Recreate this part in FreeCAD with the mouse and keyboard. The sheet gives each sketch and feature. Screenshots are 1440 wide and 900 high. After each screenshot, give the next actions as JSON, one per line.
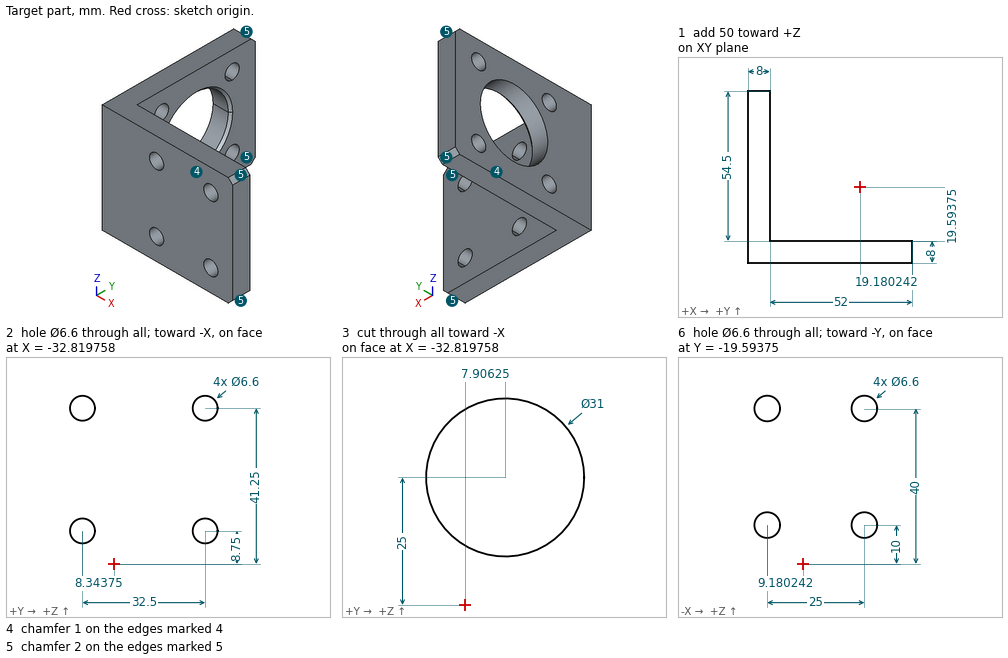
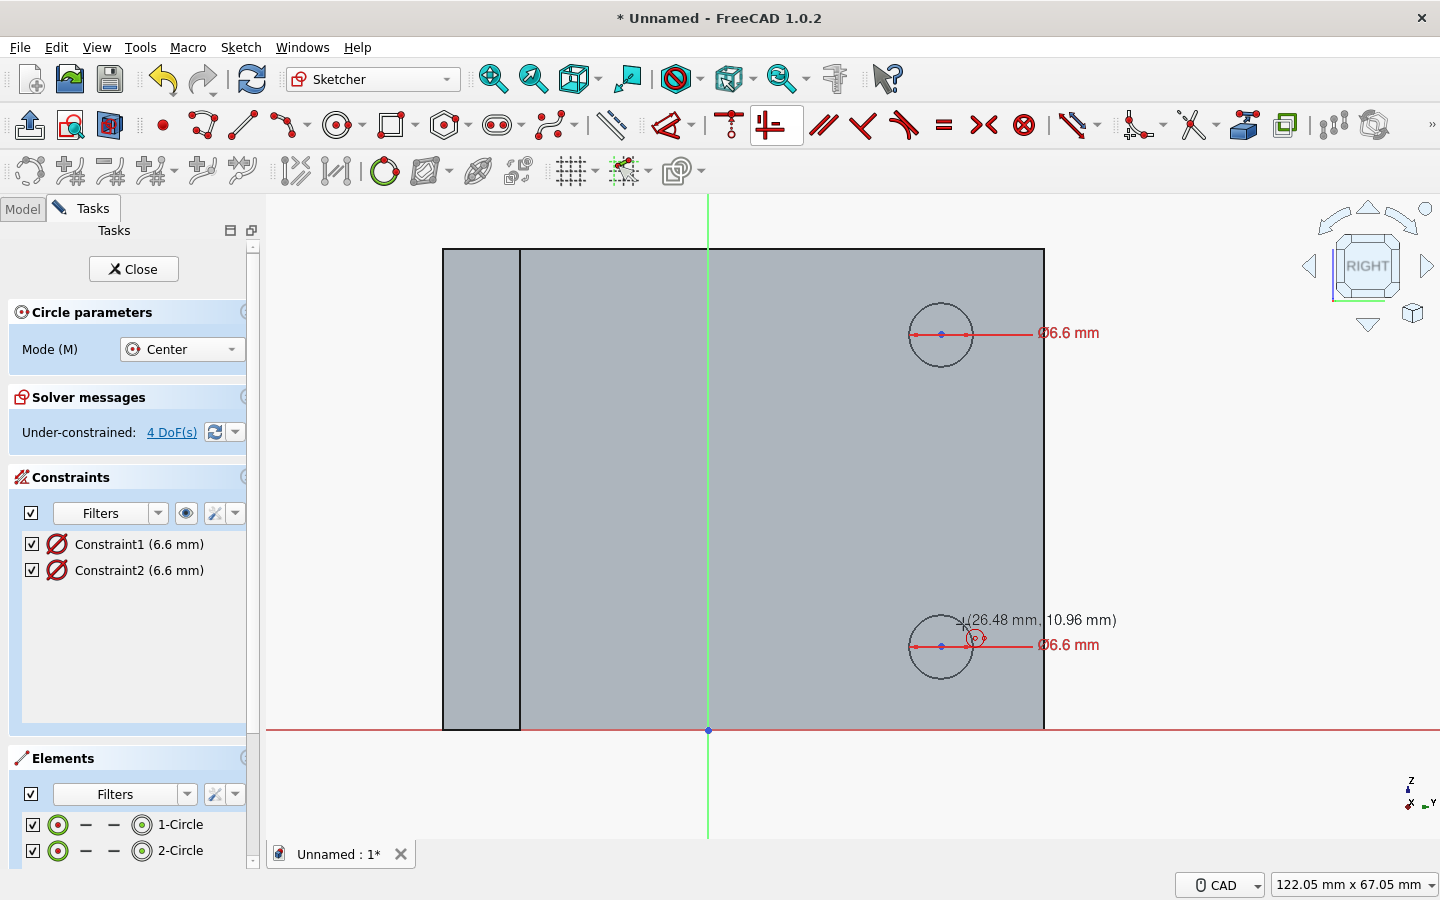
{"action": "left_click", "coordinate": [628, 646]}
{"action": "mouse_move", "coordinate": [650, 624]}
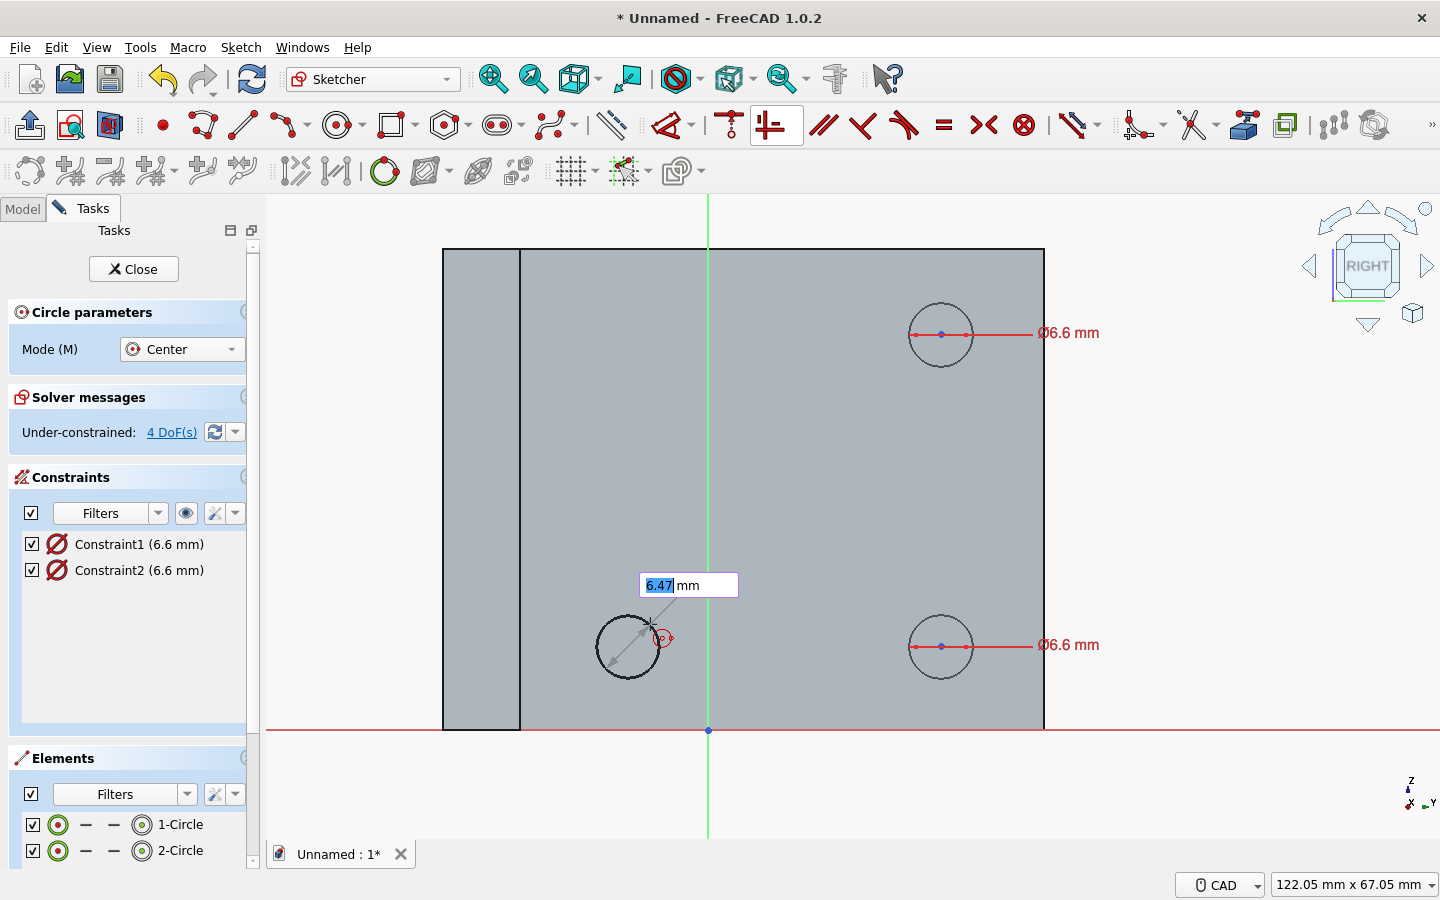
{"action": "type", "text": "6.6"}
{"action": "key", "text": "Return"}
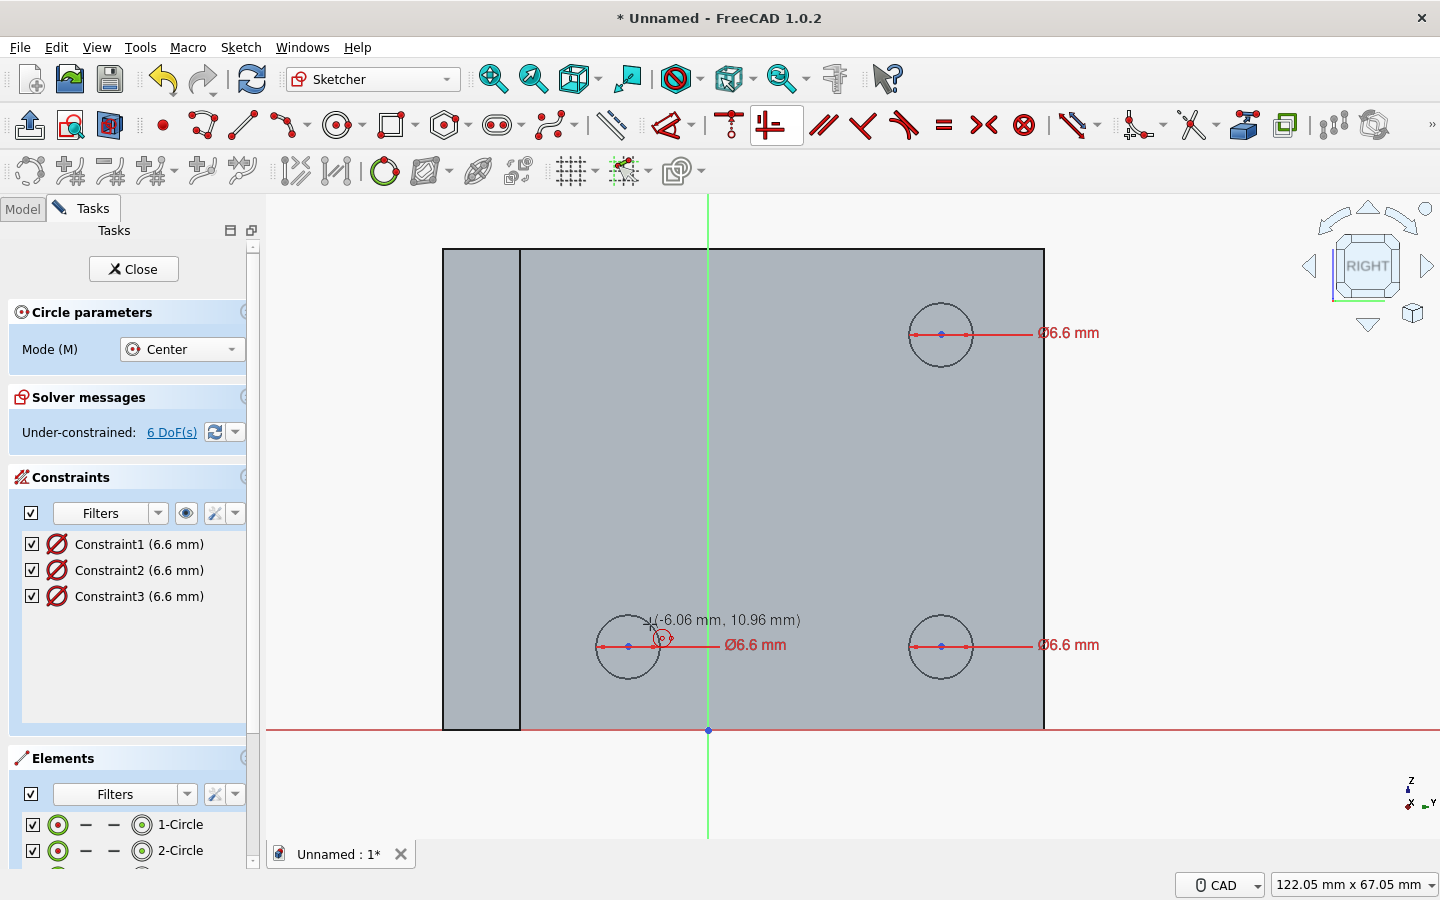
{"action": "left_click", "coordinate": [628, 334]}
{"action": "mouse_move", "coordinate": [650, 311]}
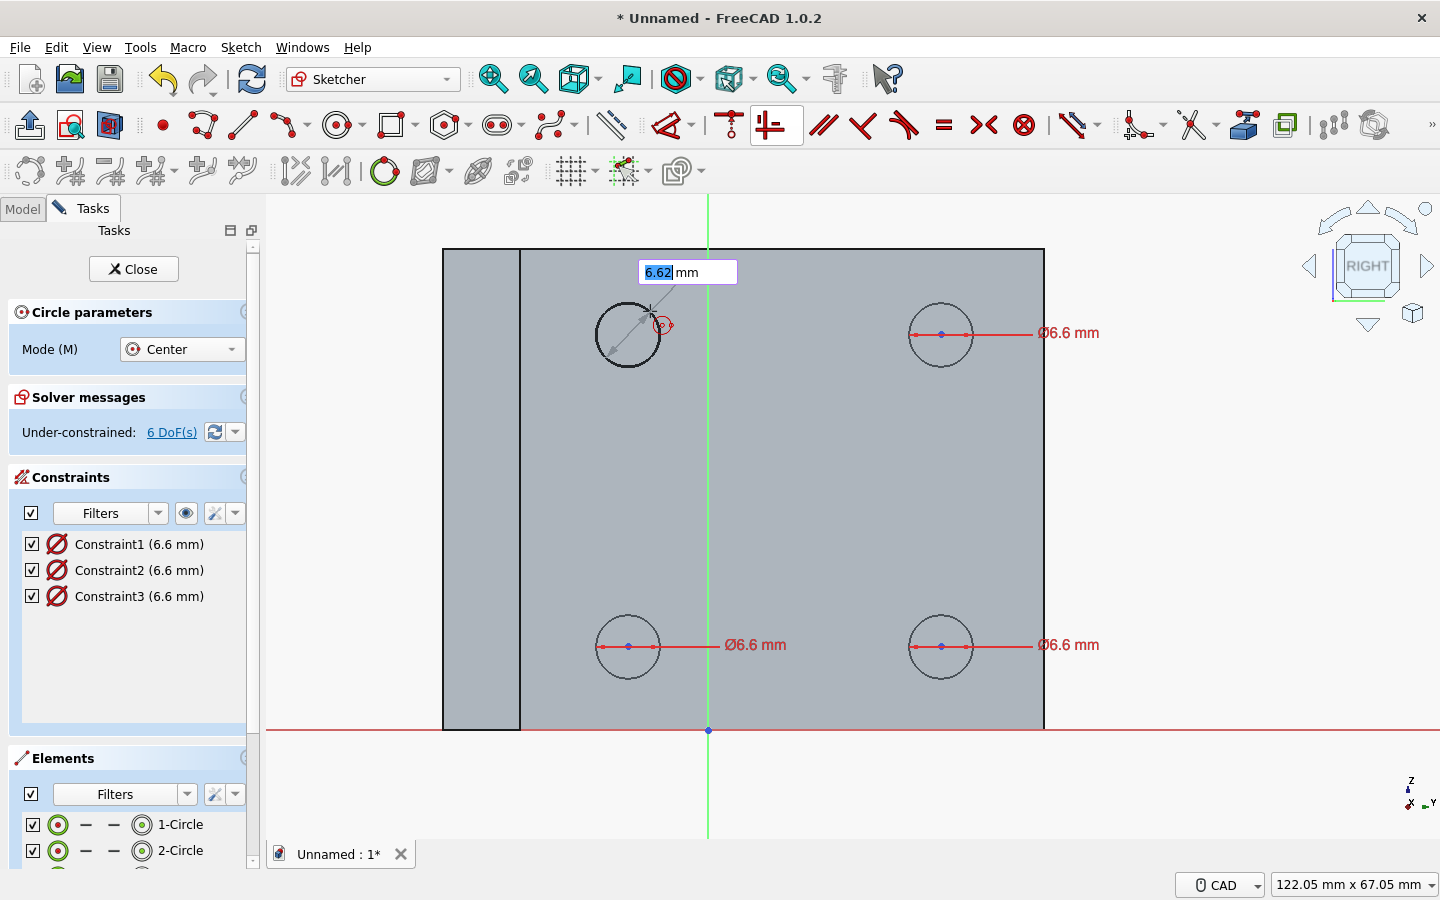
{"action": "type", "text": "6.6"}
{"action": "key", "text": "Return"}
{"action": "key", "text": "Escape"}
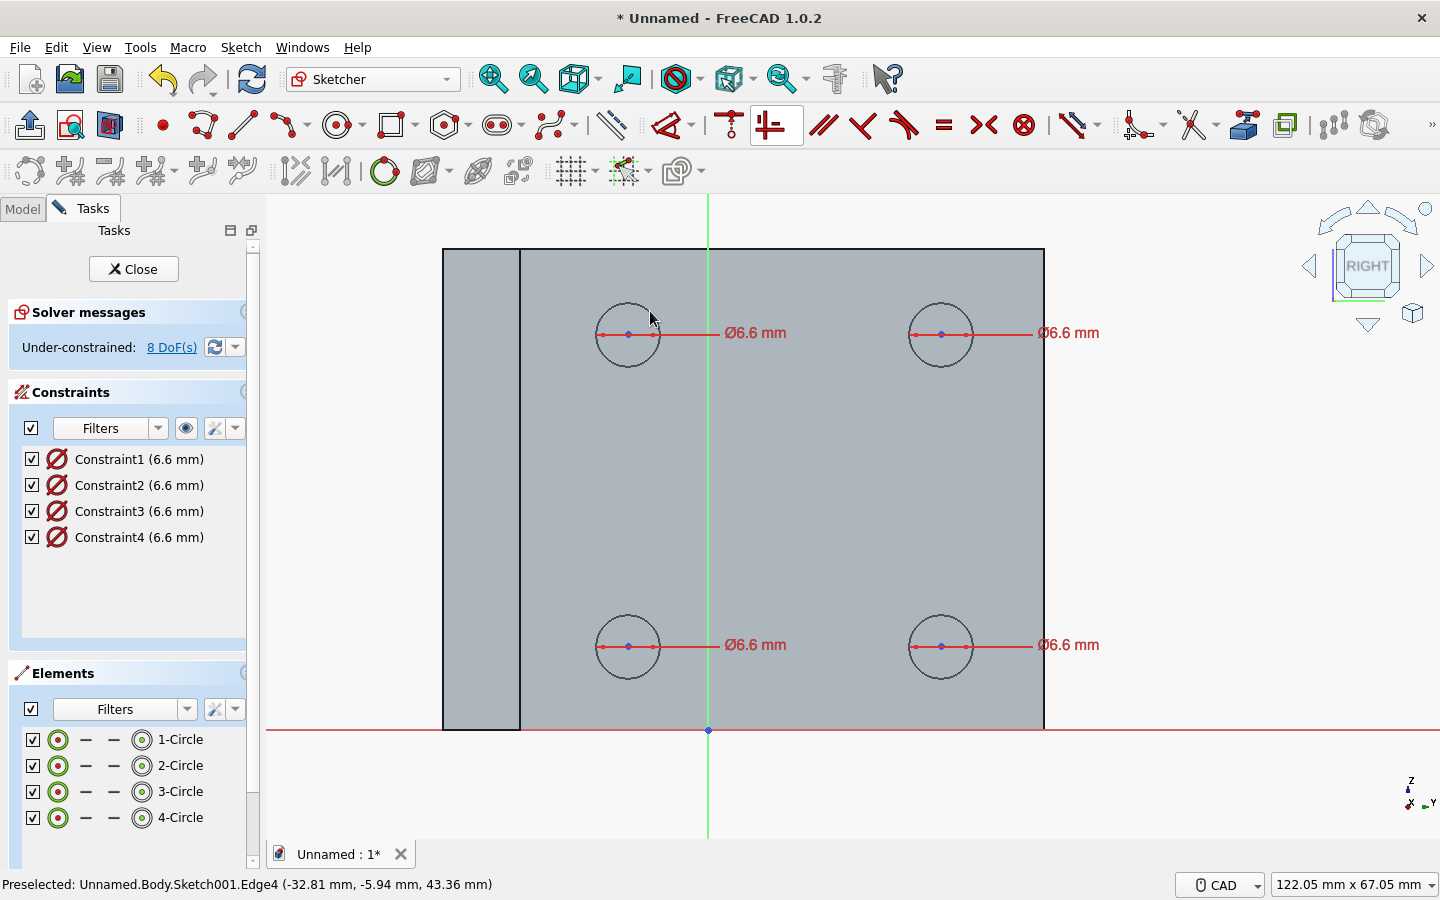
{"action": "left_click", "coordinate": [941, 335]}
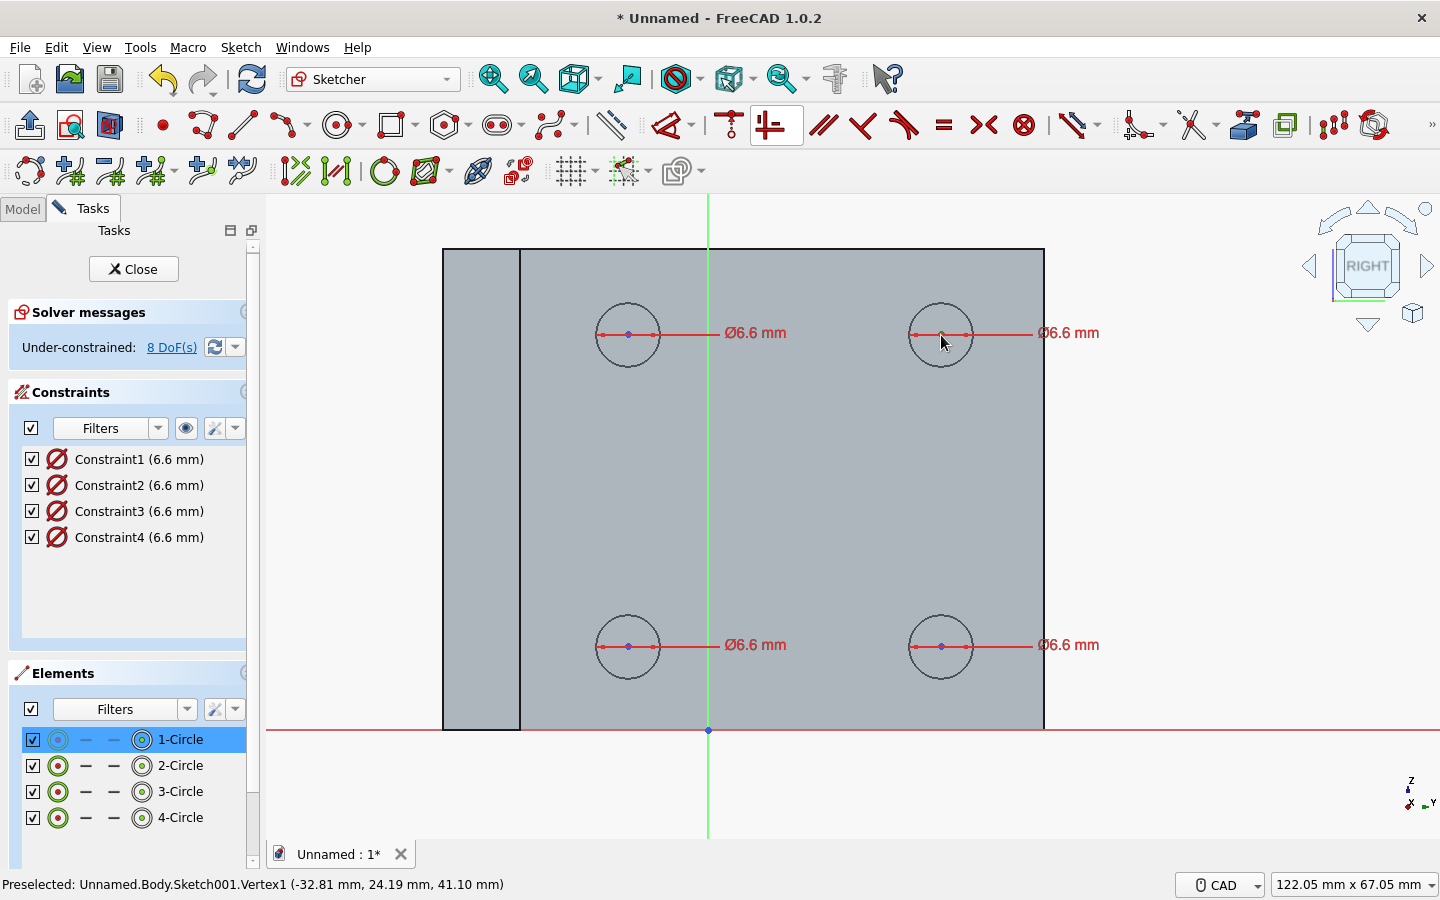
{"action": "left_click", "coordinate": [941, 647]}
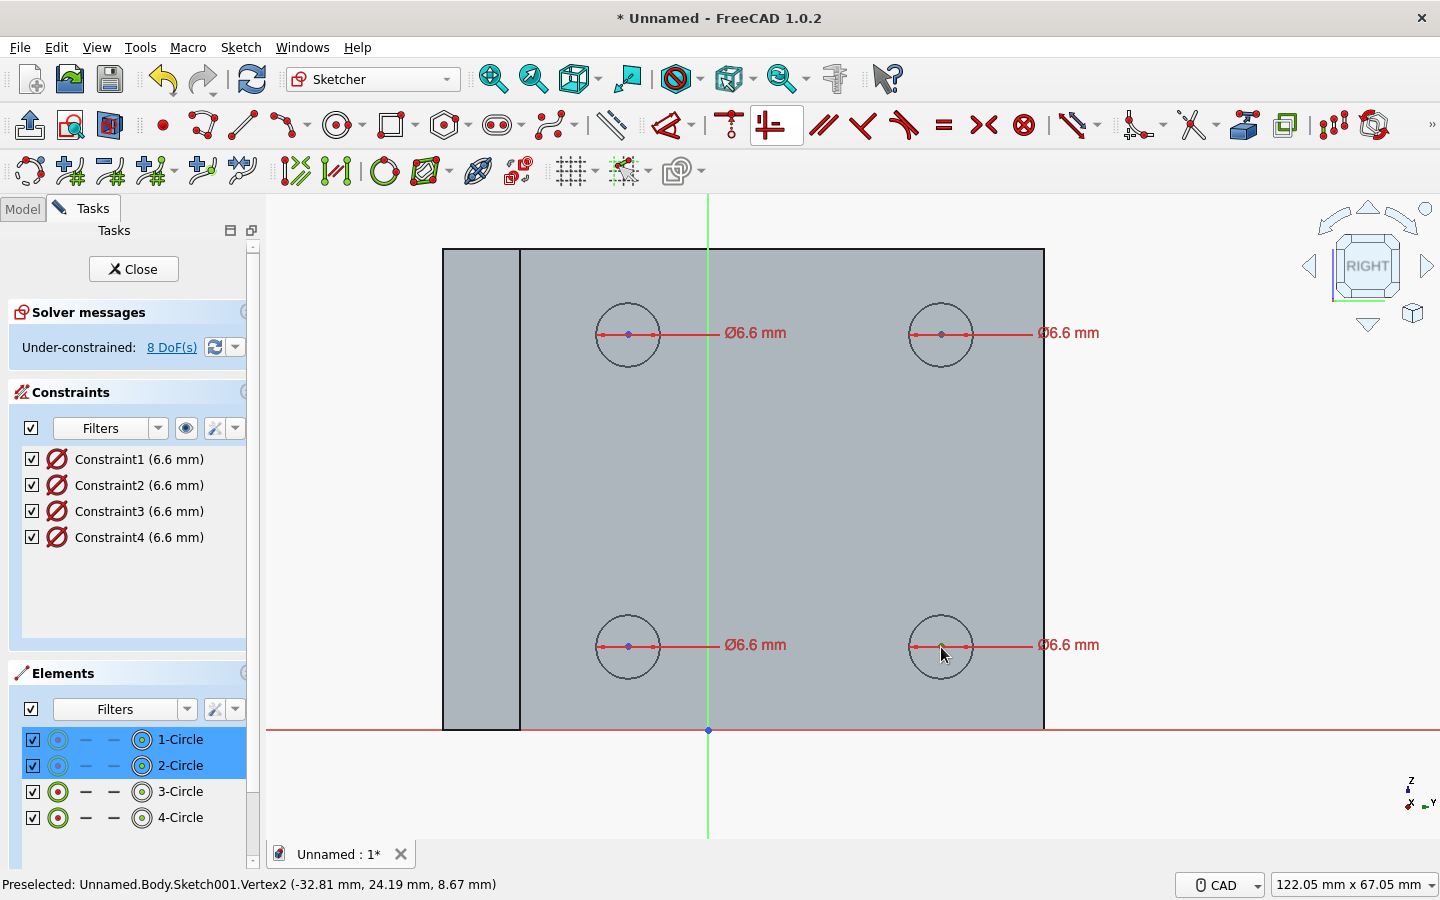
{"action": "left_click", "coordinate": [798, 126]}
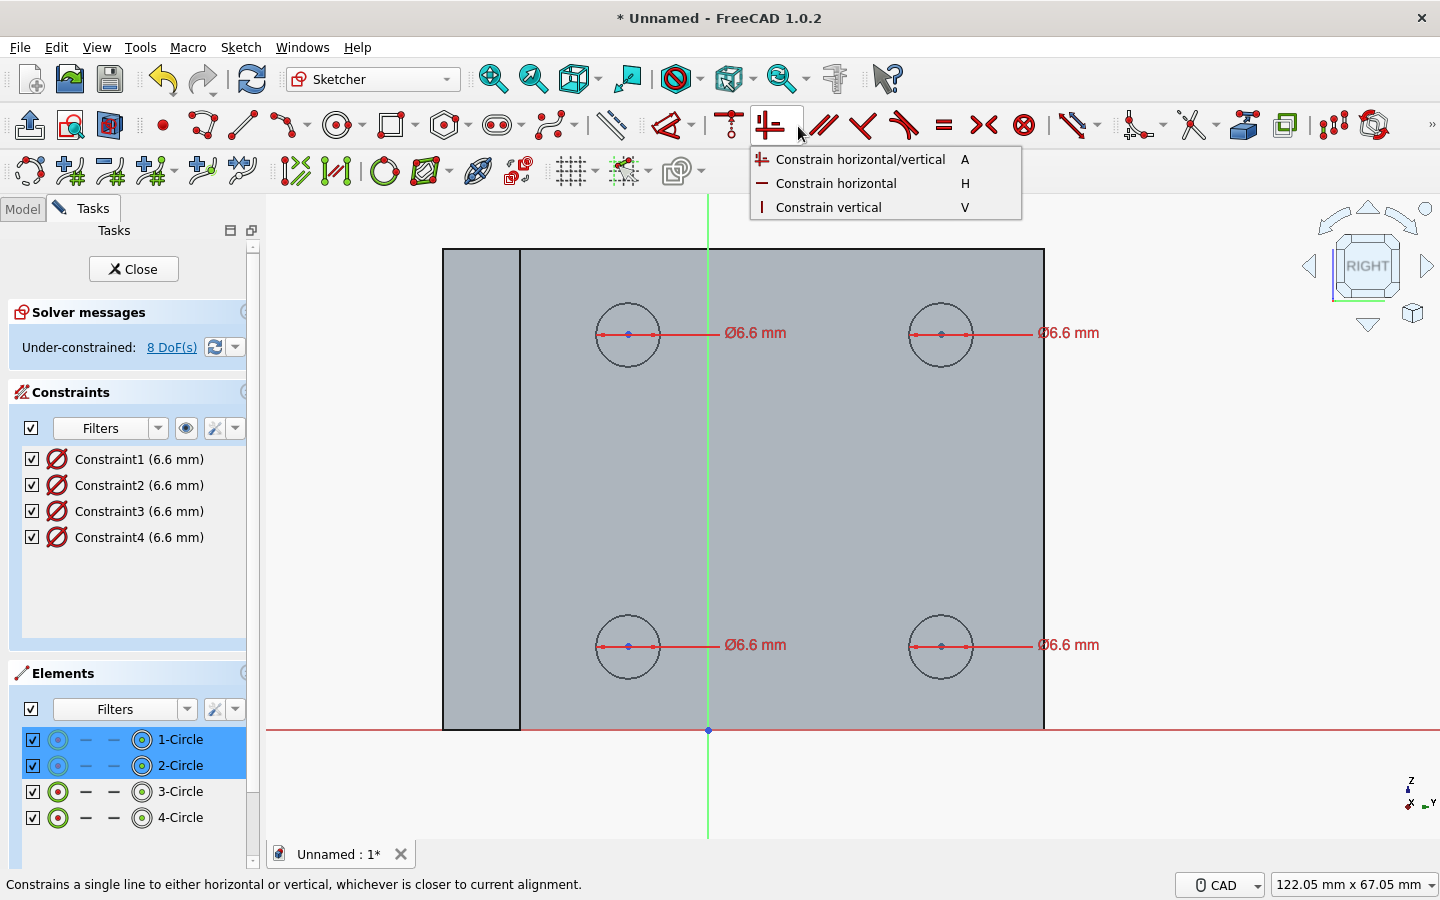
{"action": "left_click", "coordinate": [886, 207]}